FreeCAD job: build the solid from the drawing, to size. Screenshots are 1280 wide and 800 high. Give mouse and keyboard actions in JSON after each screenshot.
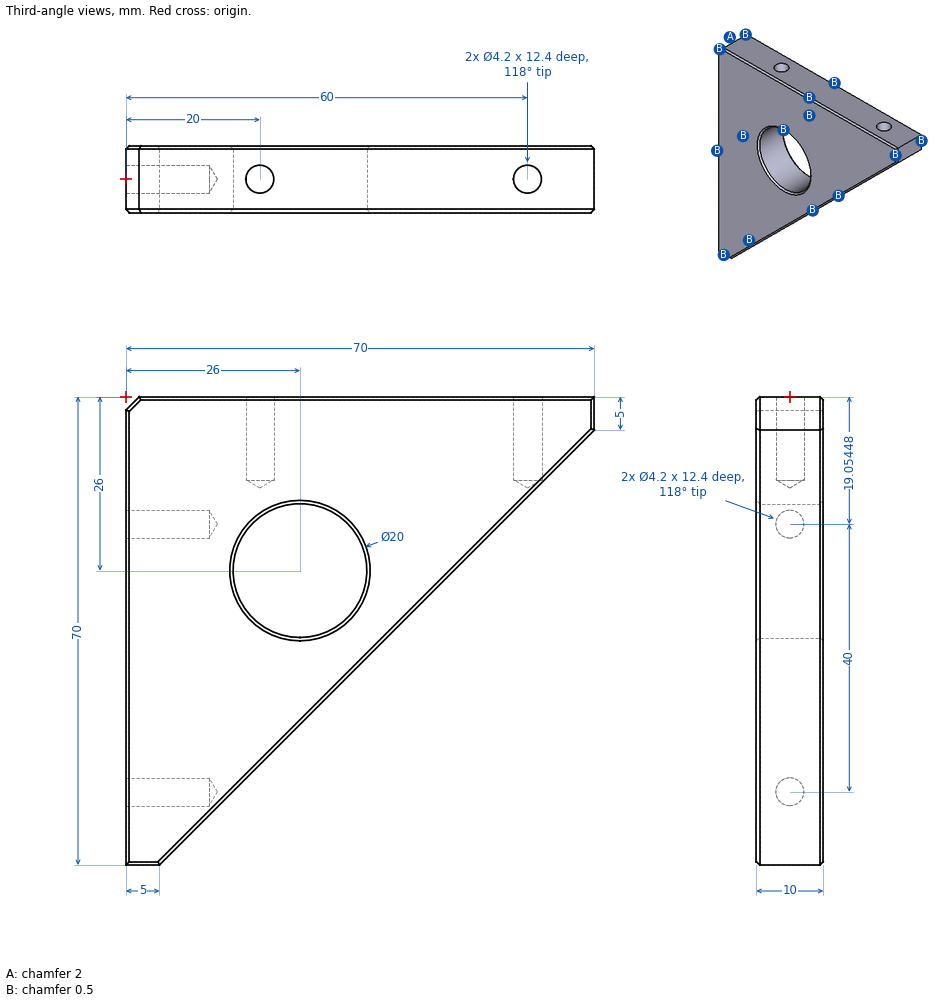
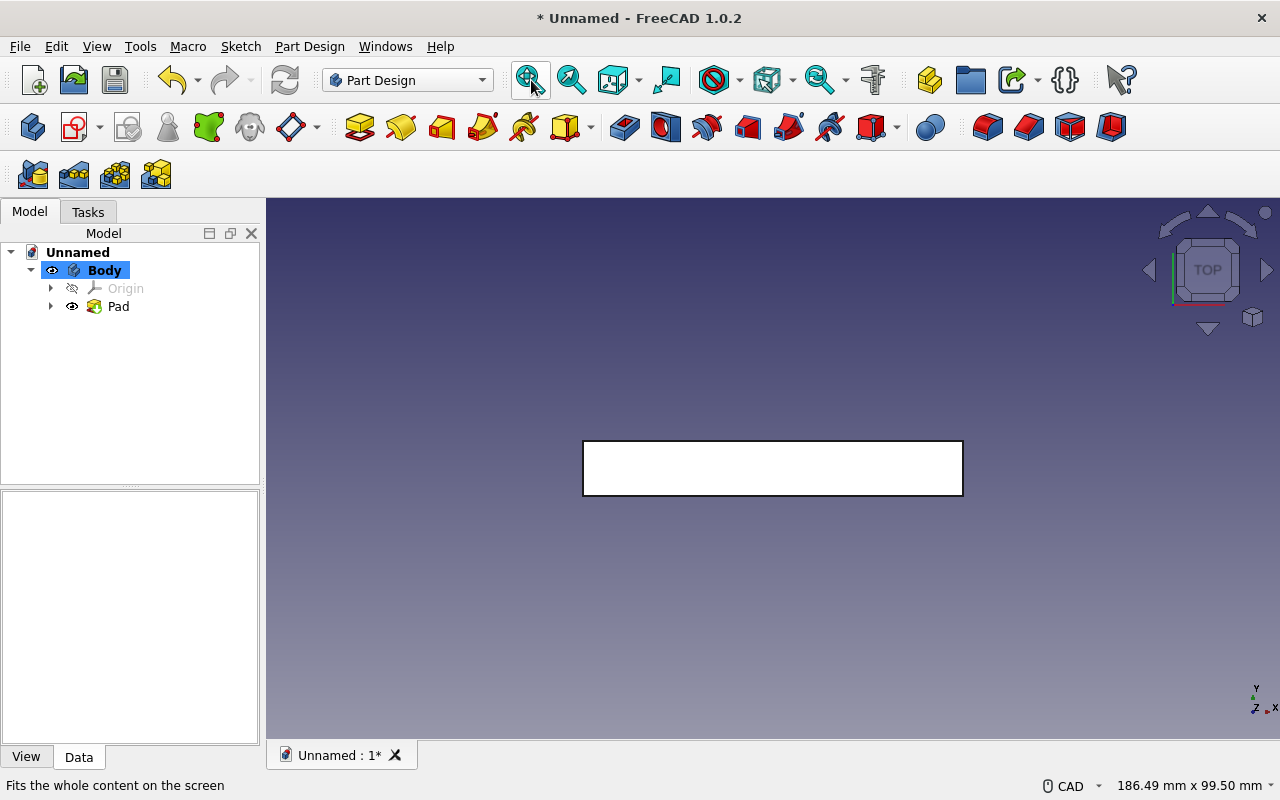
{"action": "left_click", "coordinate": [583, 468]}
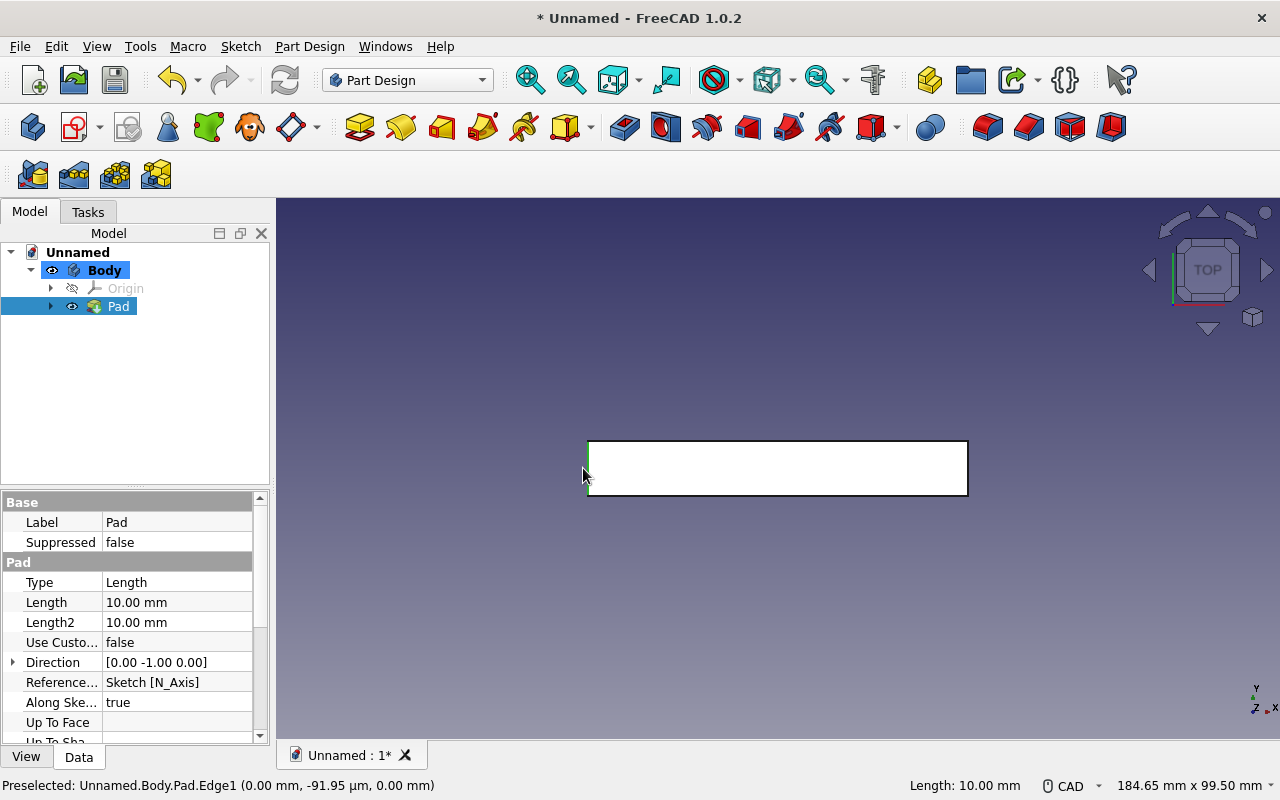
{"action": "left_click", "coordinate": [1029, 128]}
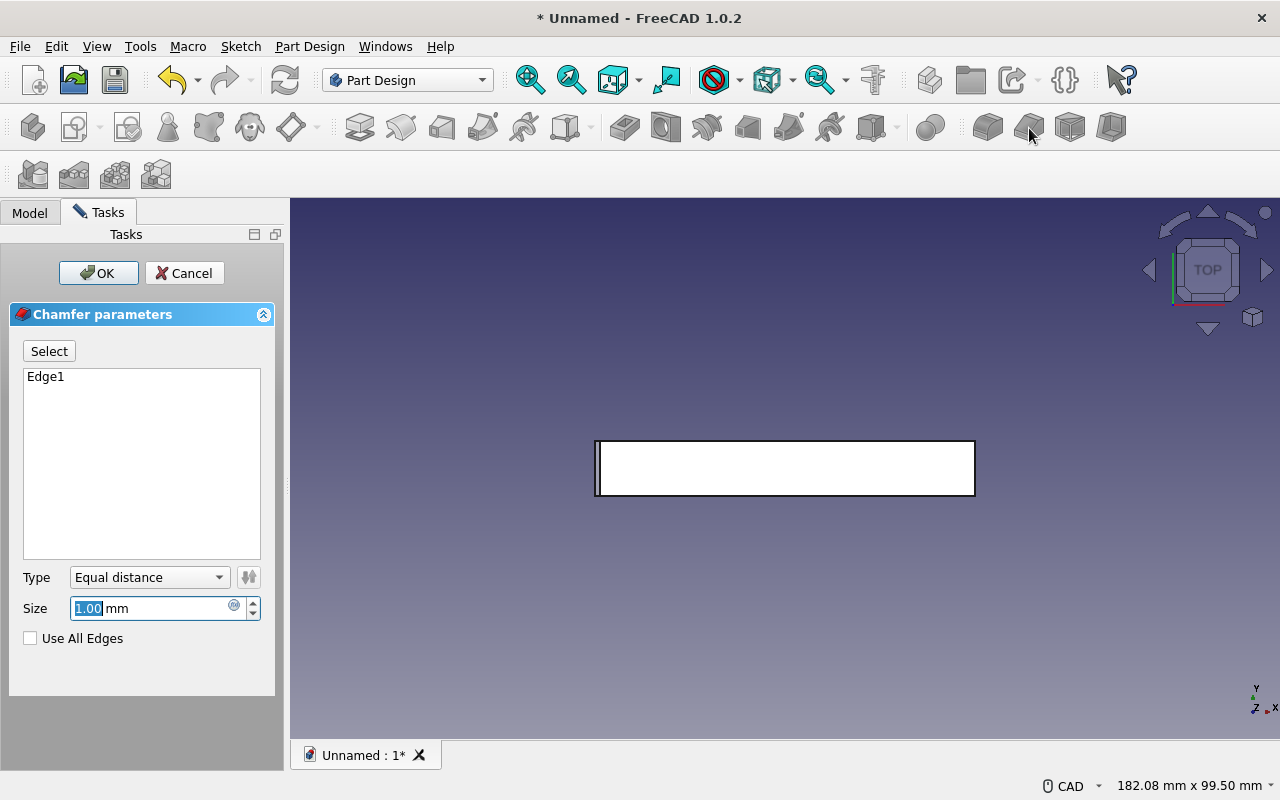
{"action": "type", "text": "2"}
{"action": "key", "text": "Tab"}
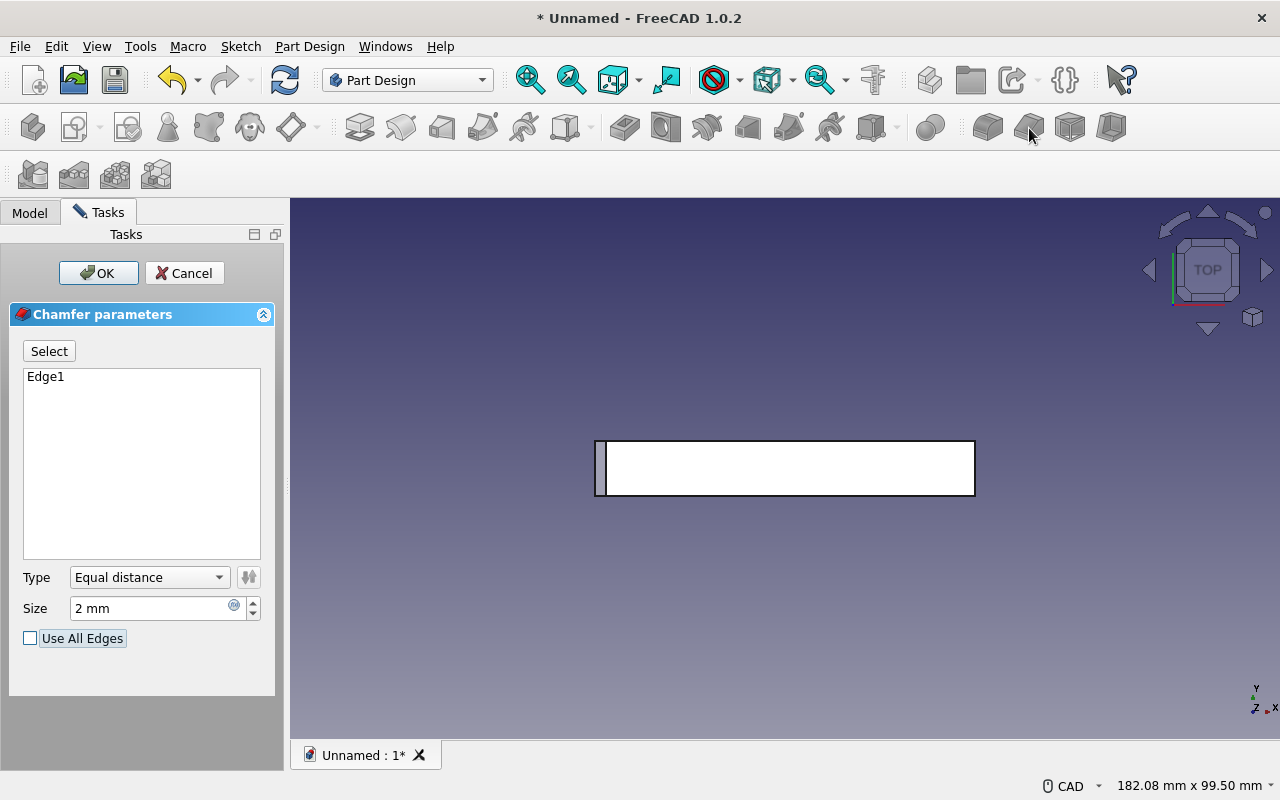
{"action": "left_click", "coordinate": [99, 273]}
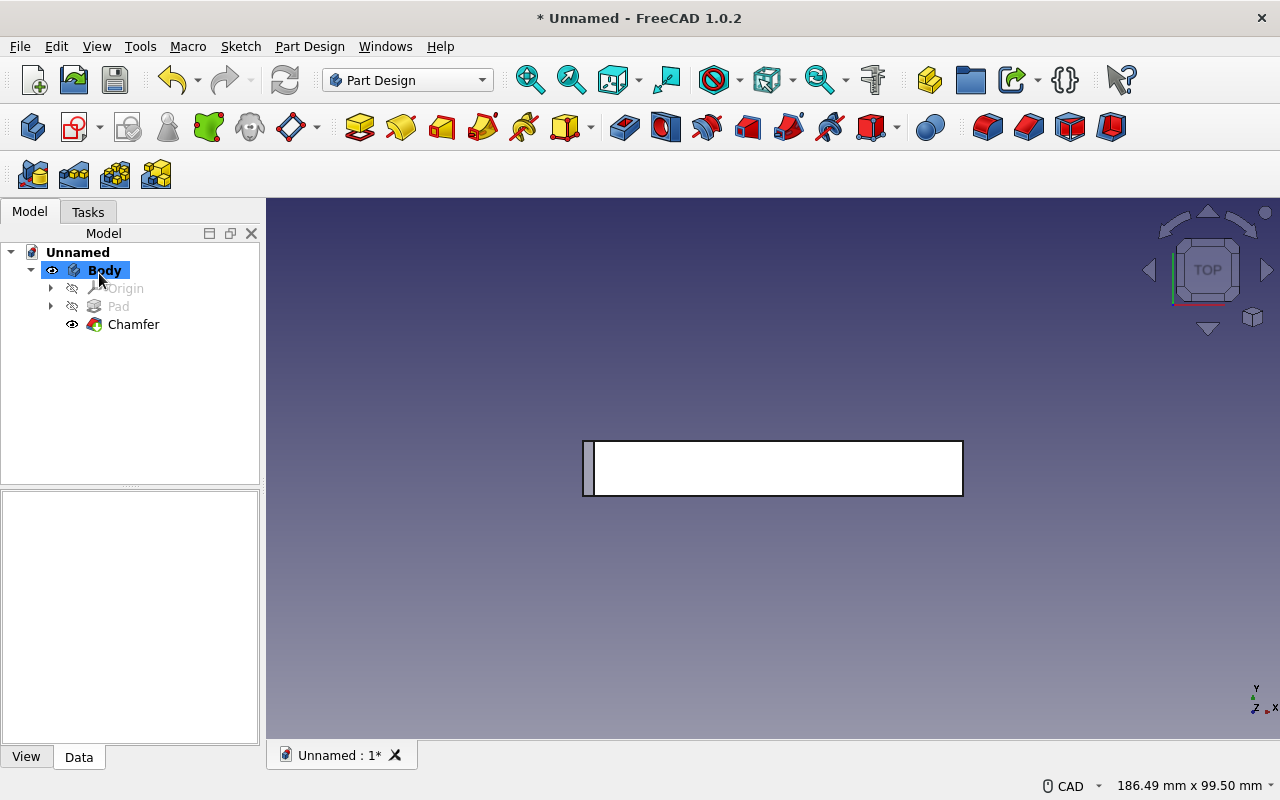
{"action": "left_click", "coordinate": [531, 80]}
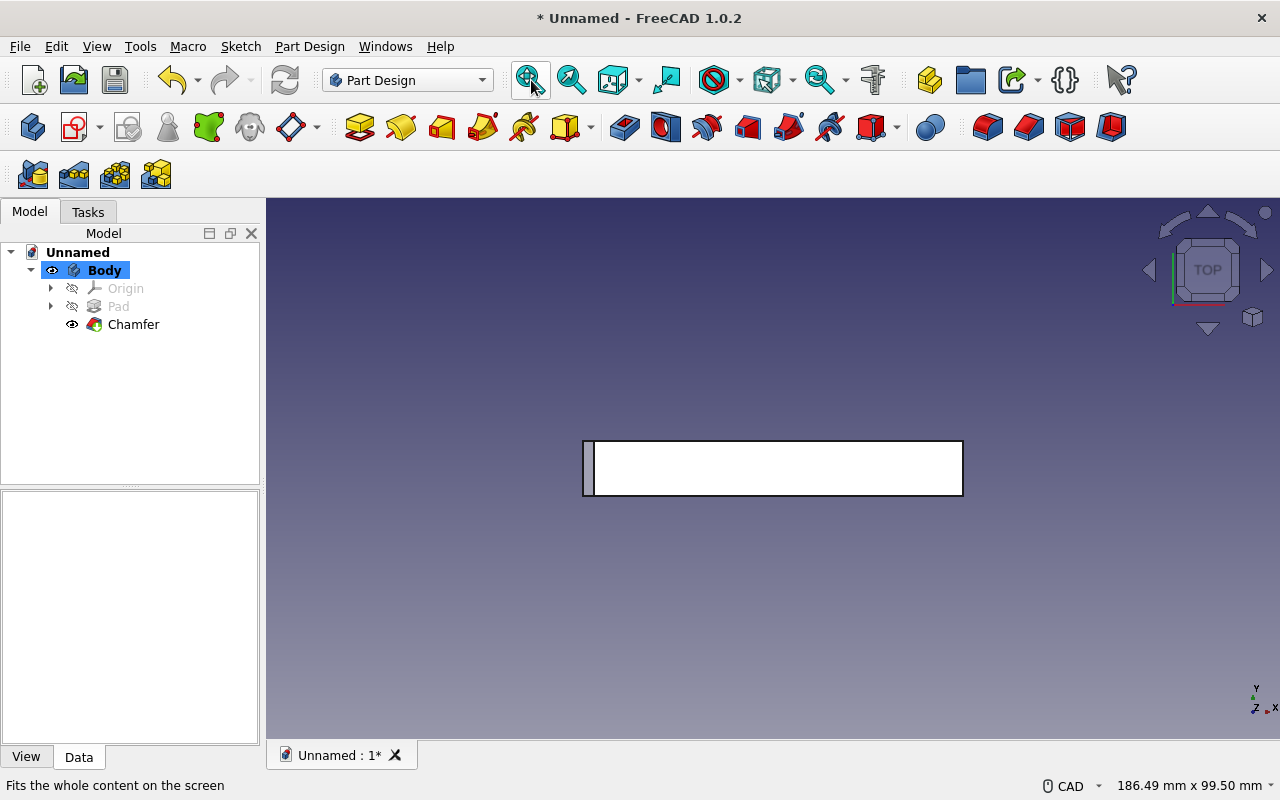
{"action": "left_click", "coordinate": [74, 128]}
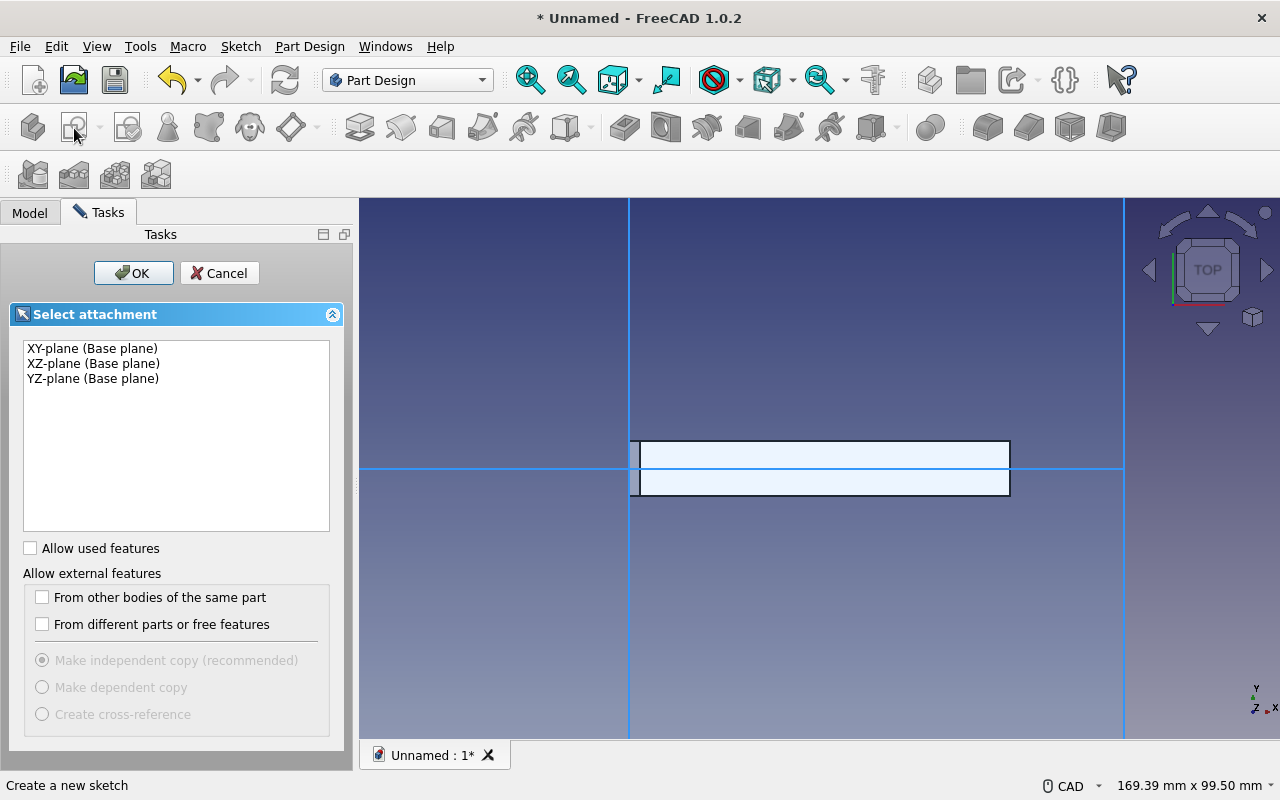
{"action": "left_click", "coordinate": [84, 348]}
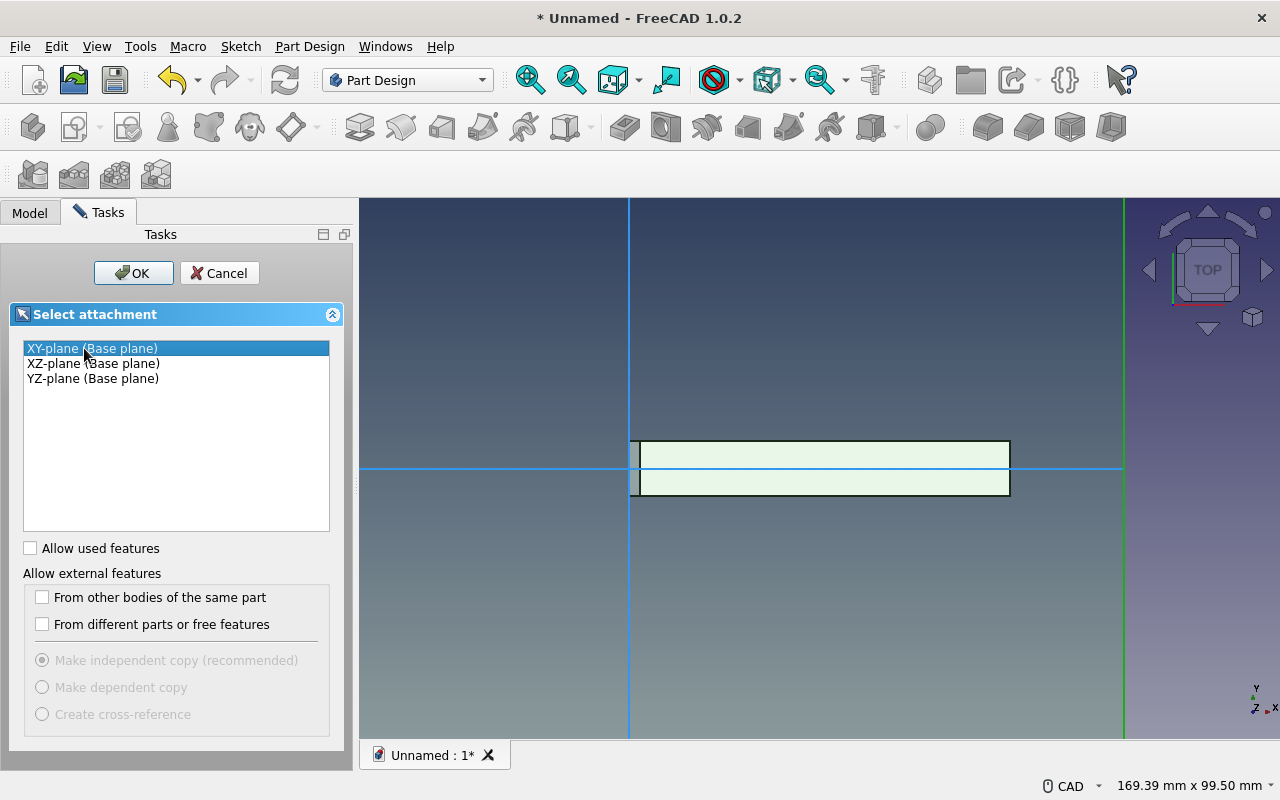
{"action": "left_click", "coordinate": [134, 273]}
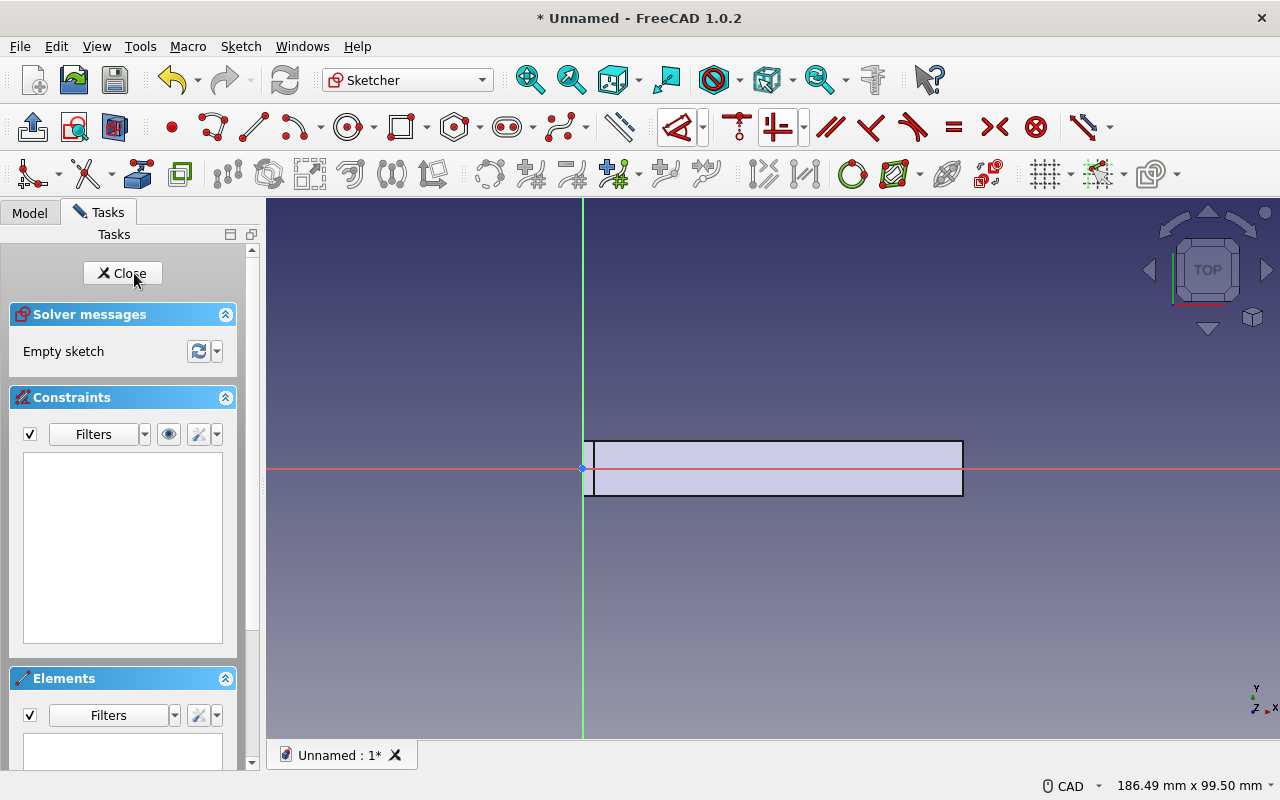
{"action": "scroll", "coordinate": [809, 469], "scroll_direction": "up", "scroll_amount": 3}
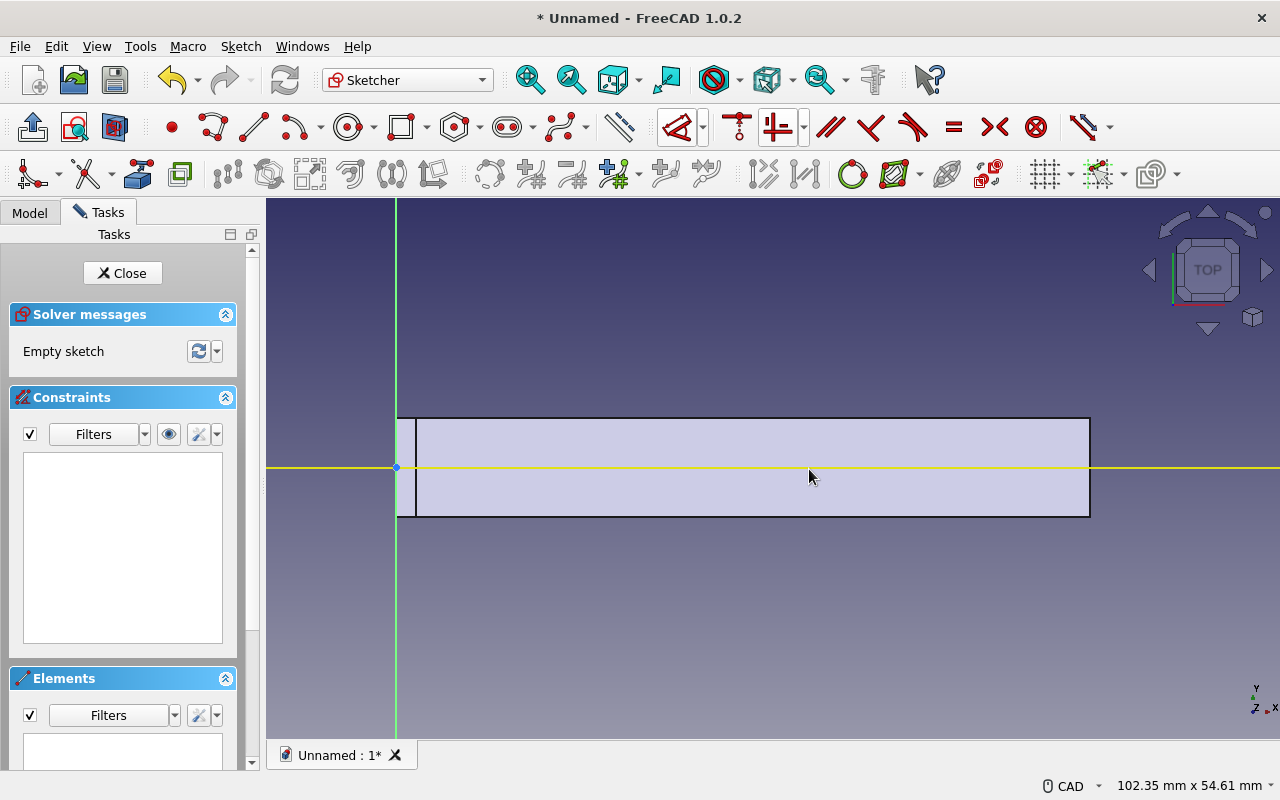
{"action": "left_click", "coordinate": [348, 128]}